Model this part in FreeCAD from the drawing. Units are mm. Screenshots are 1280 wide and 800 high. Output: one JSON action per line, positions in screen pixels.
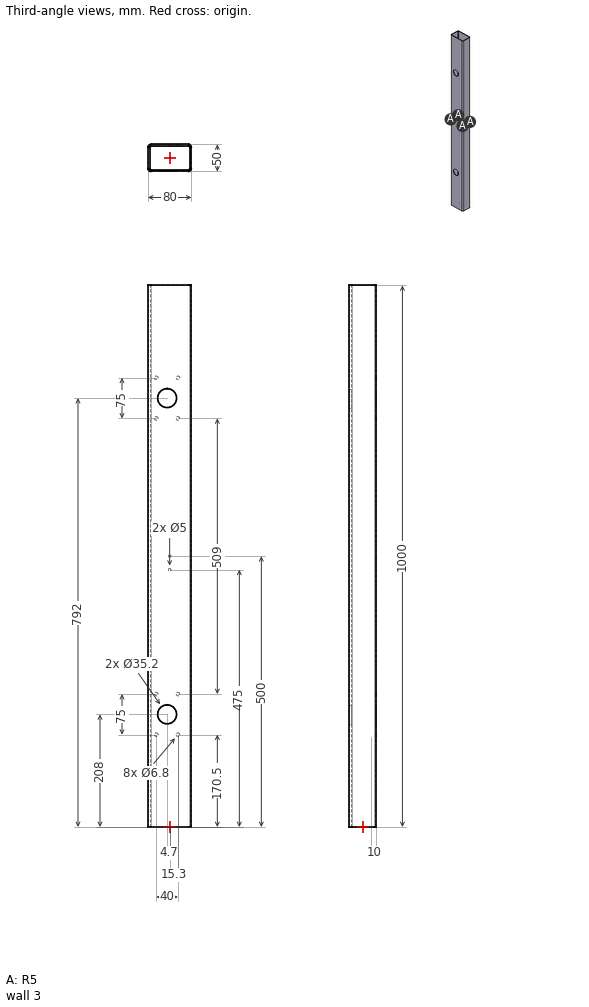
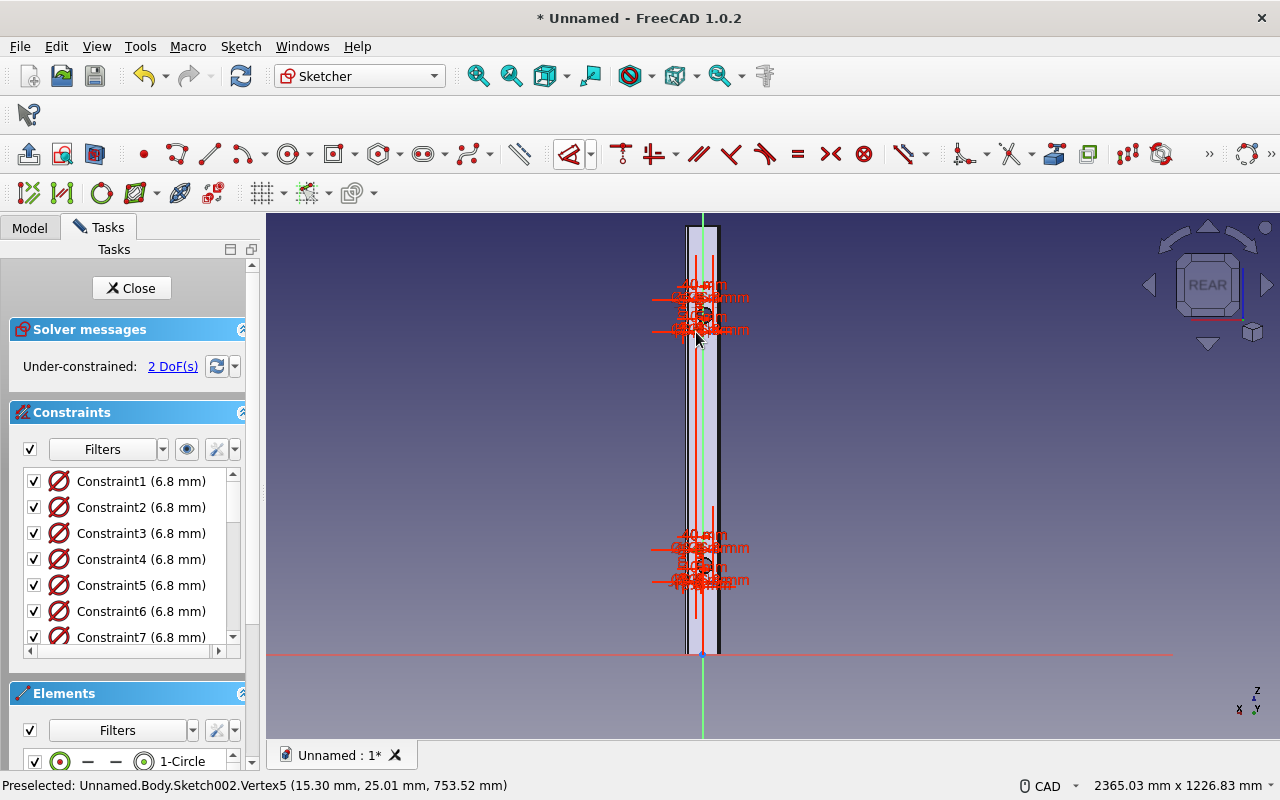
{"action": "key", "text": "i"}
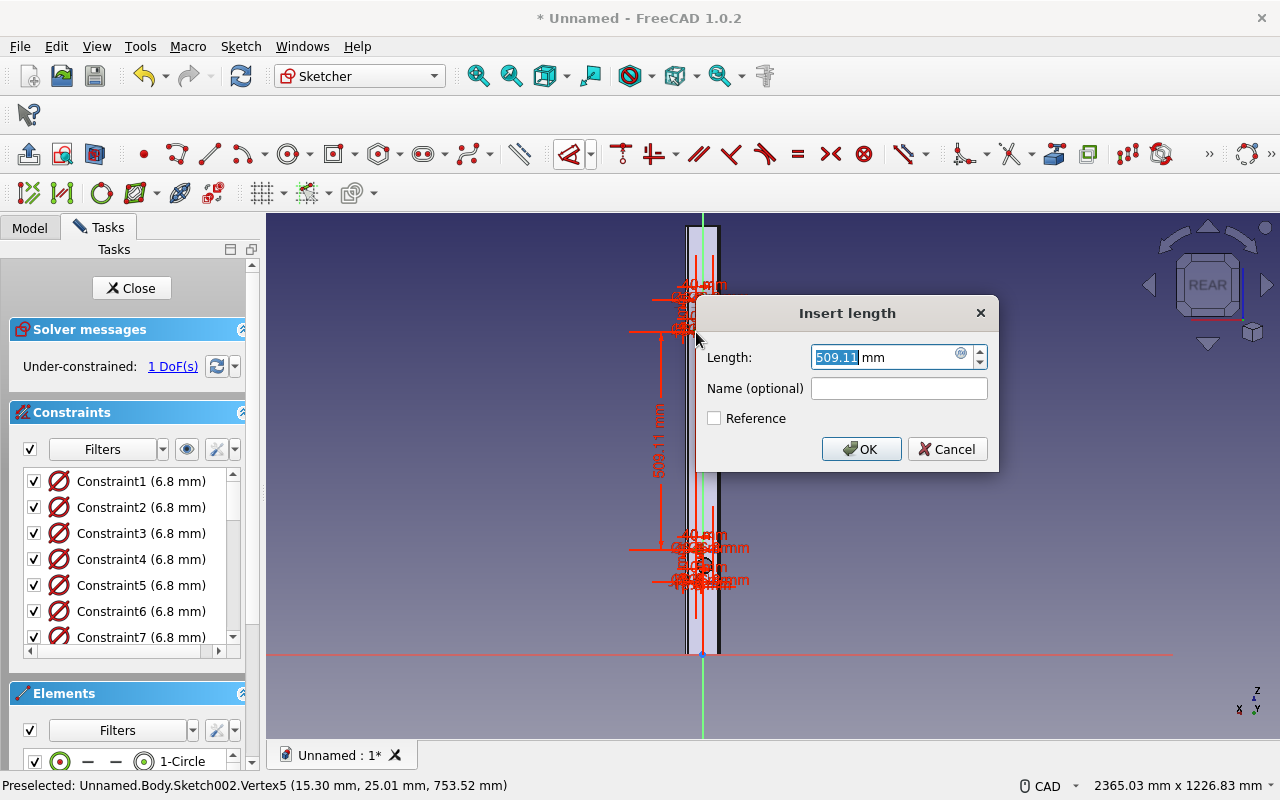
{"action": "type", "text": "509"}
{"action": "key", "text": "Return"}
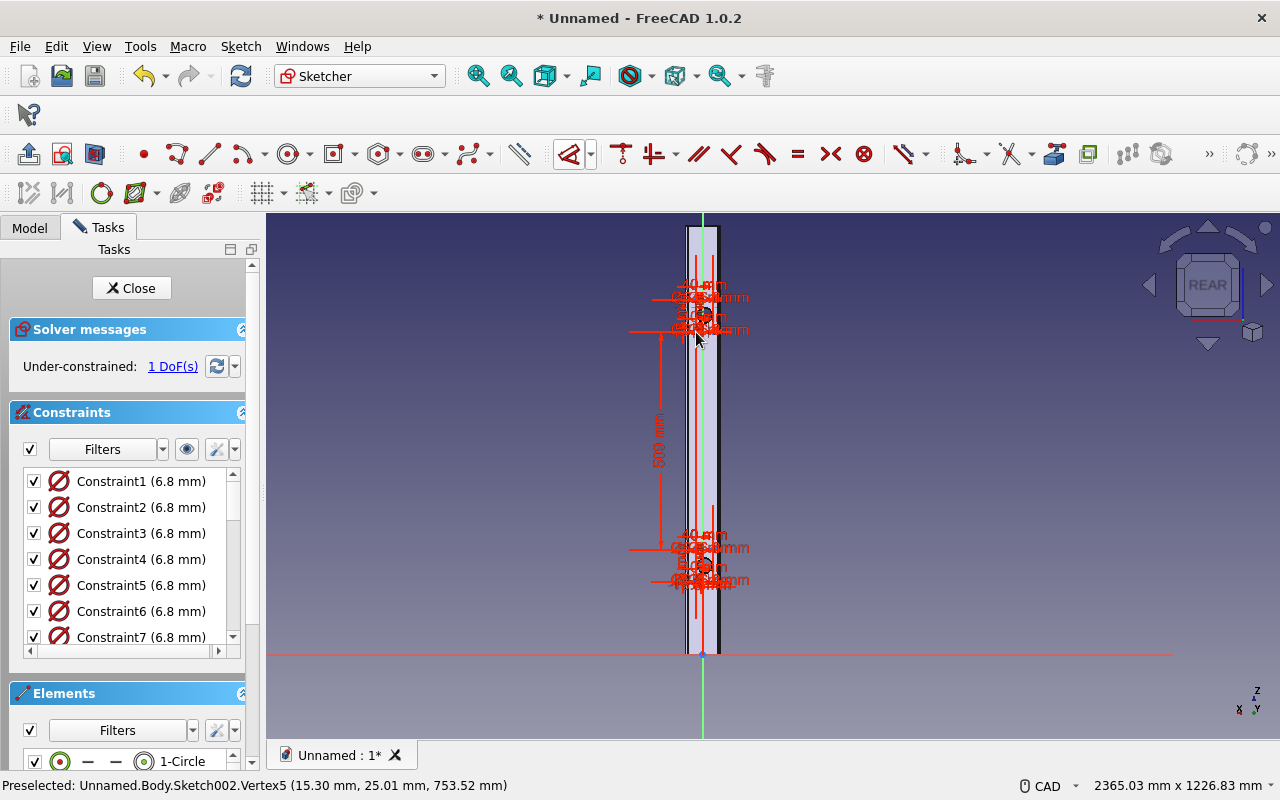
{"action": "left_click", "coordinate": [696, 582]}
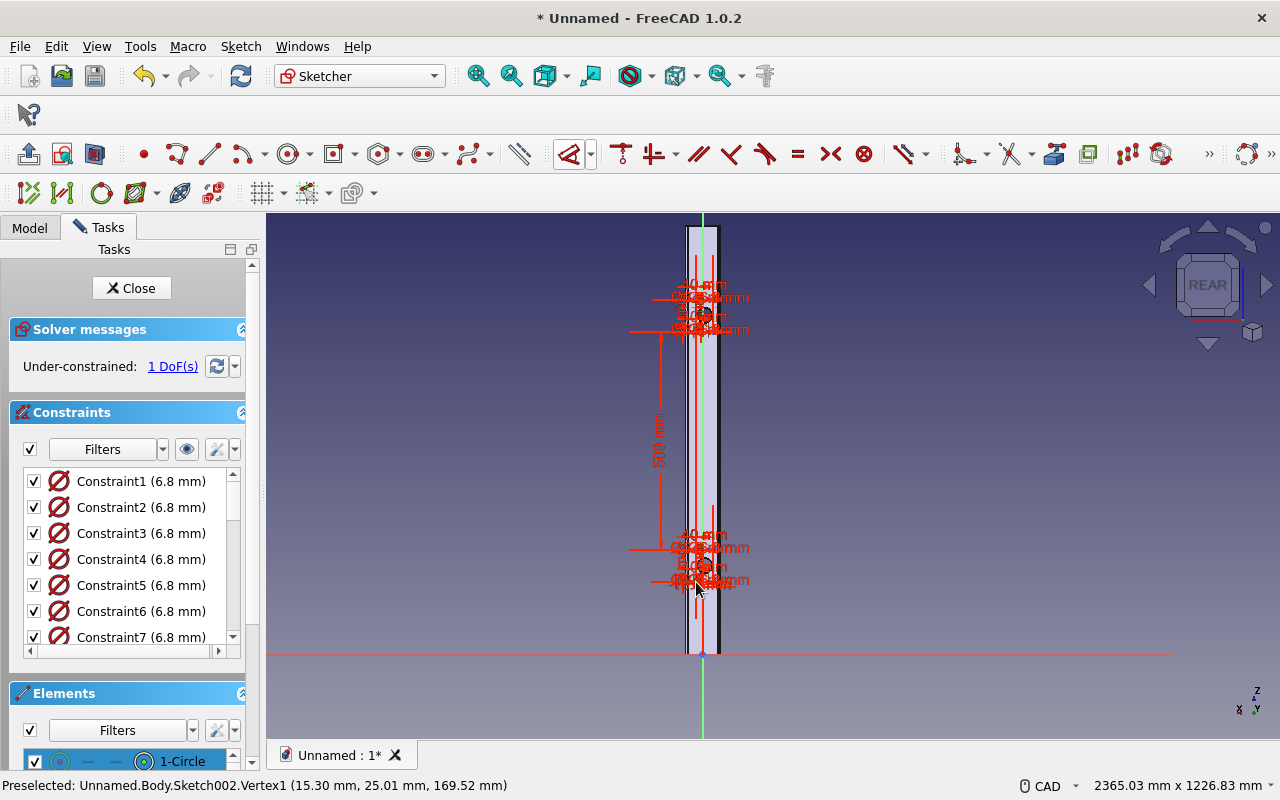
{"action": "left_click", "coordinate": [590, 154]}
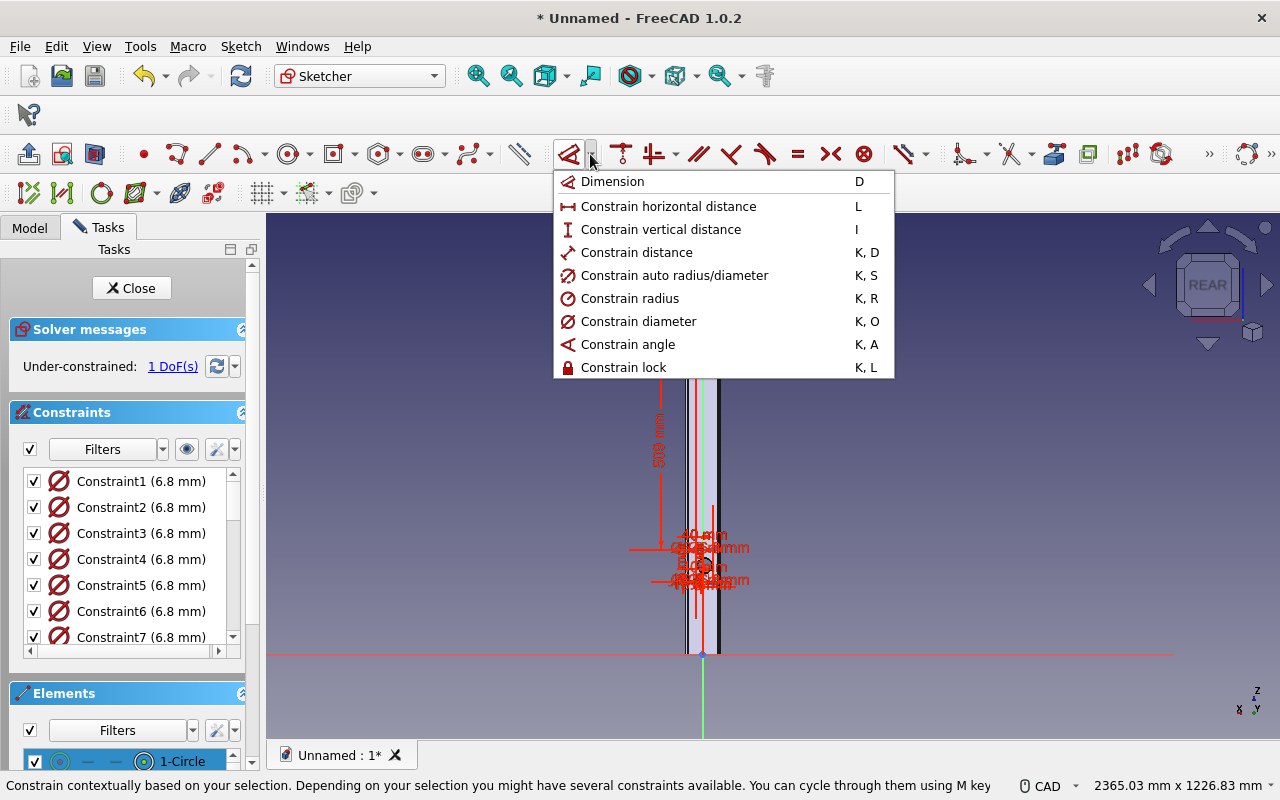
{"action": "left_click", "coordinate": [724, 230]}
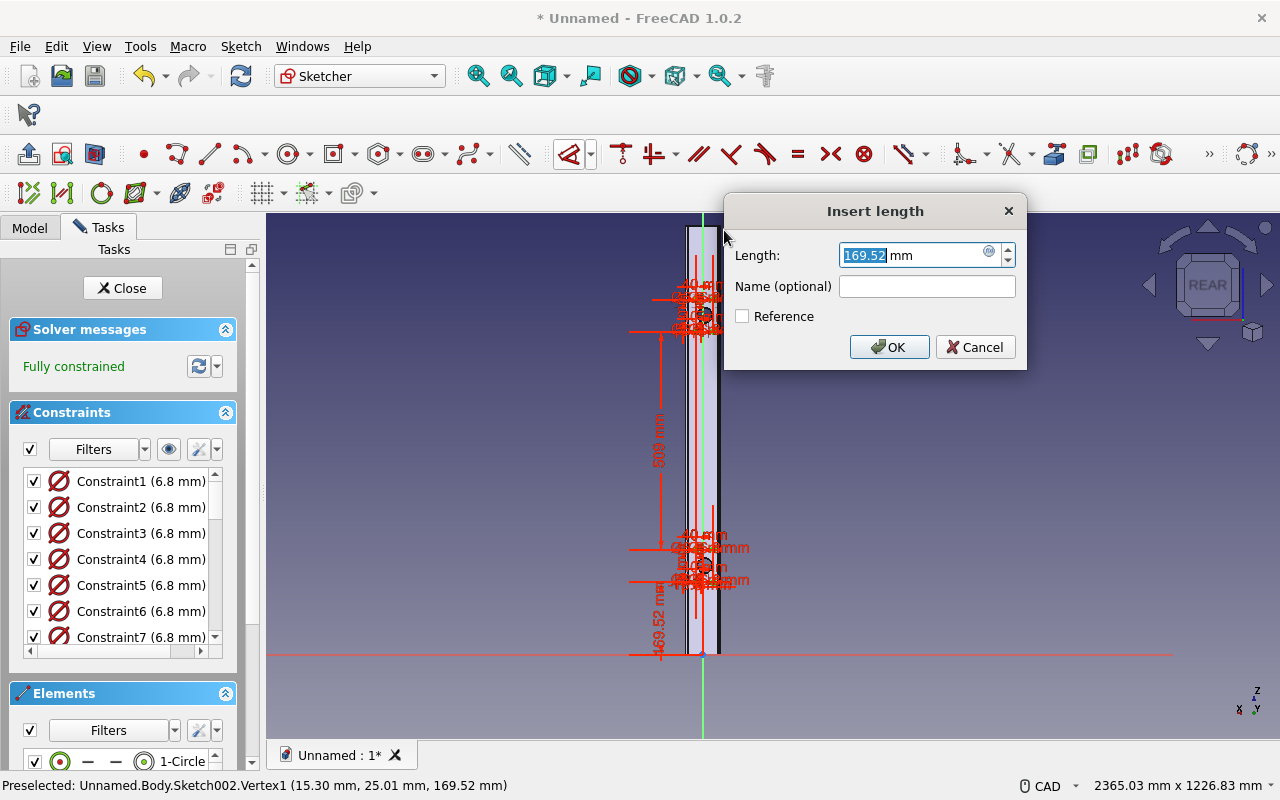
{"action": "type", "text": "170.5"}
{"action": "key", "text": "Return"}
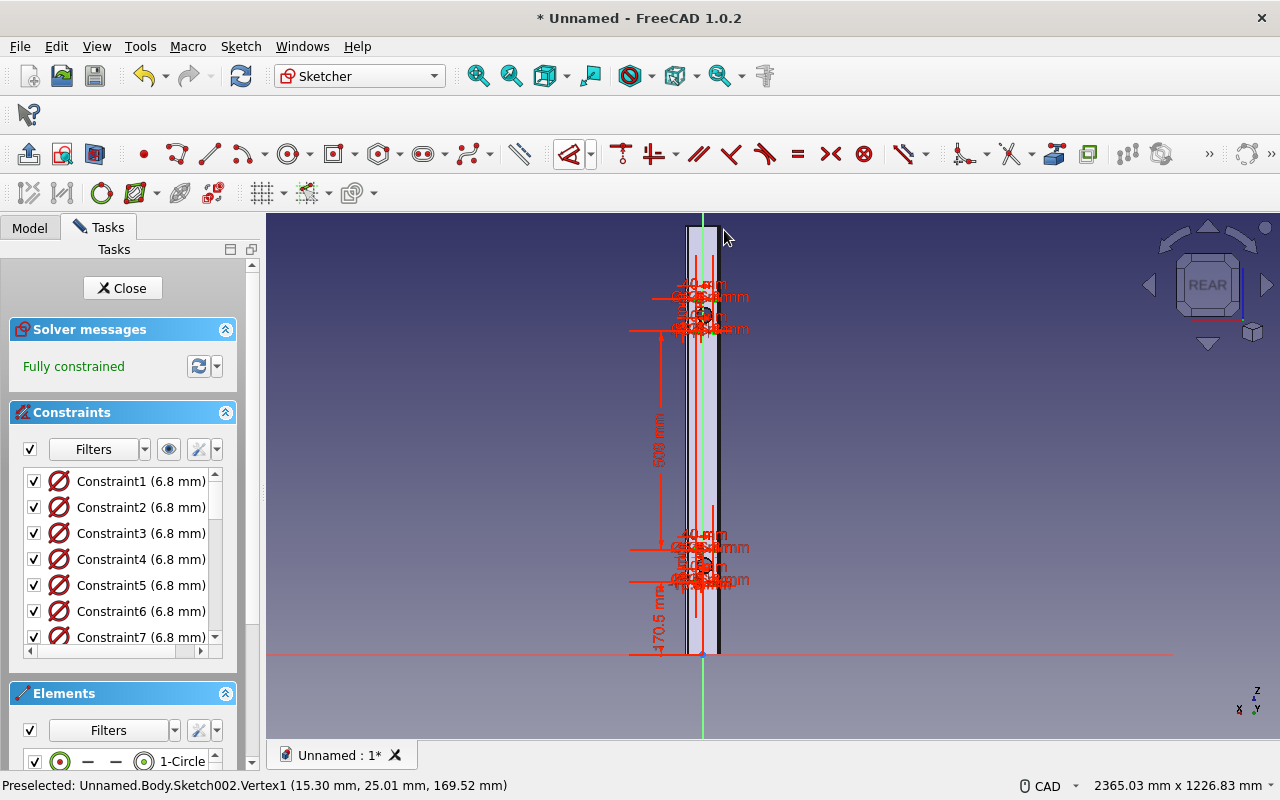
{"action": "left_click", "coordinate": [123, 288]}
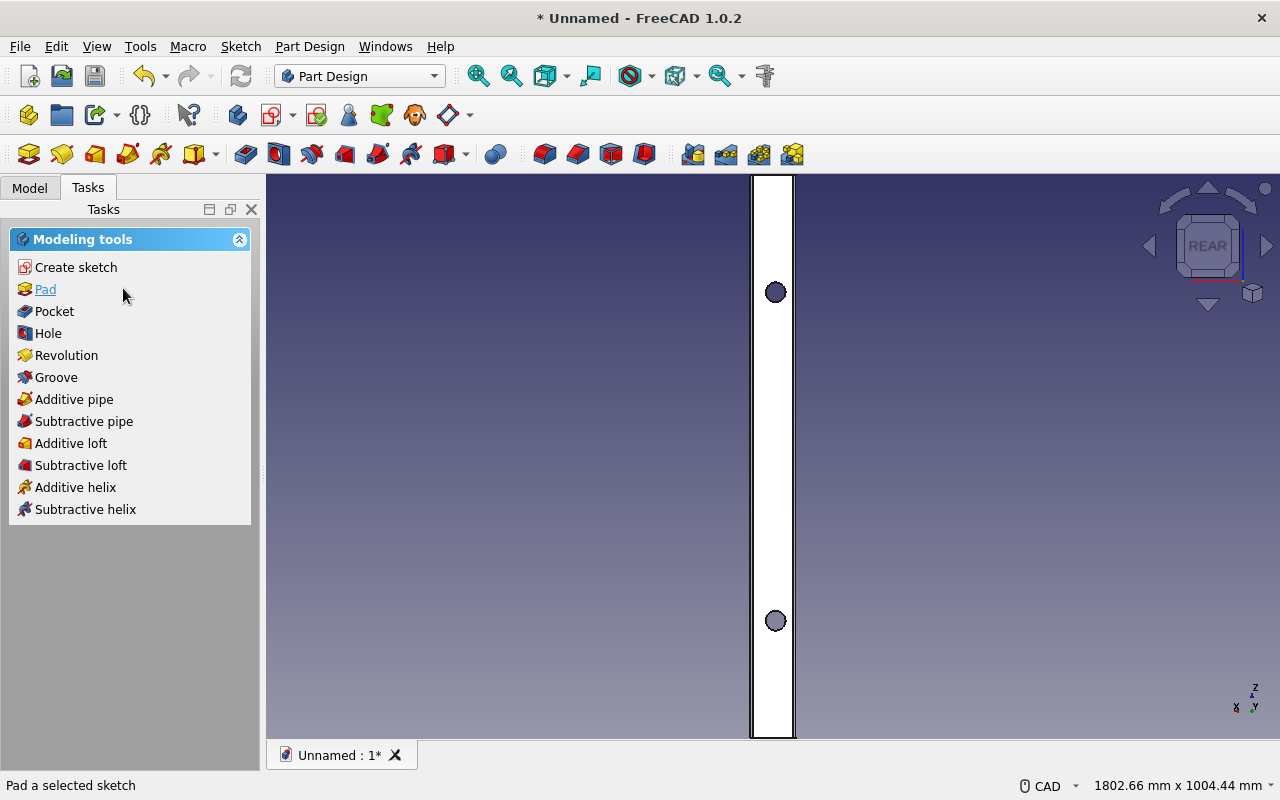
{"action": "left_click", "coordinate": [246, 154]}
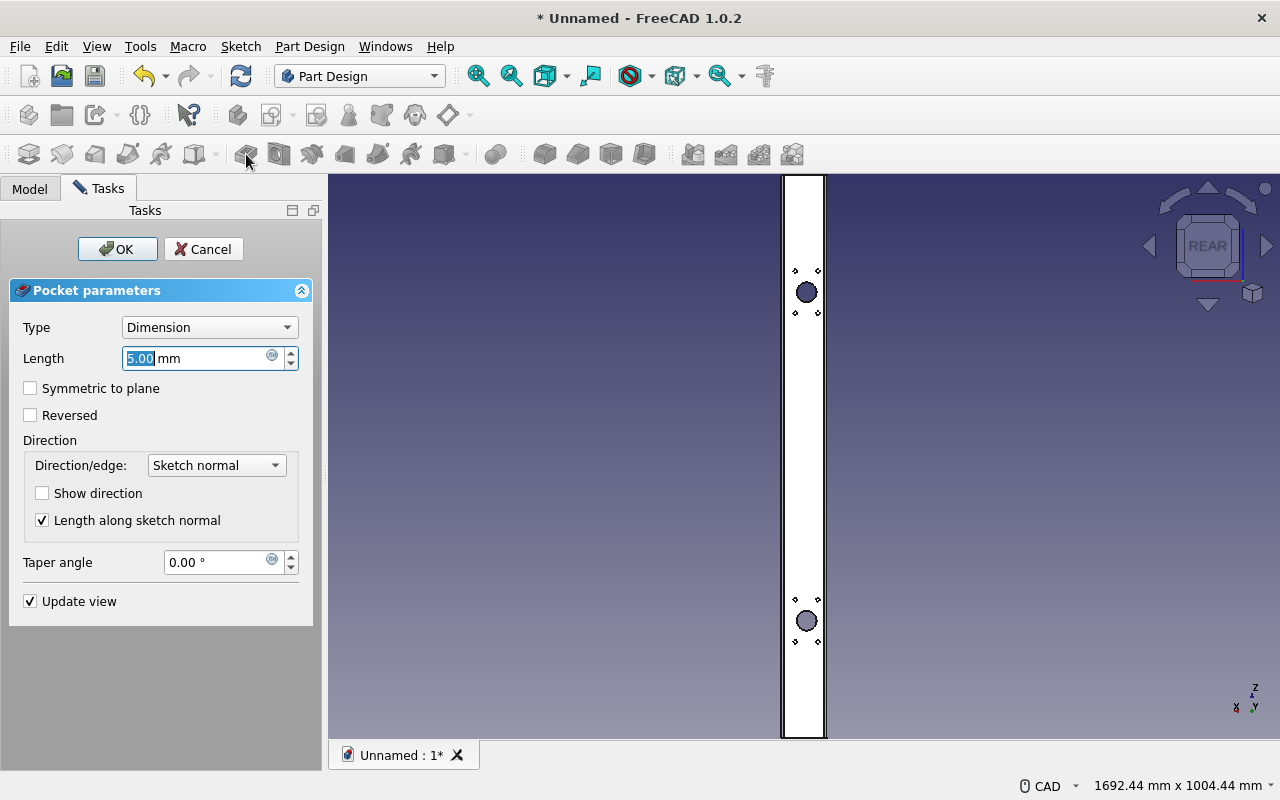
{"action": "type", "text": "10"}
{"action": "key", "text": "Tab"}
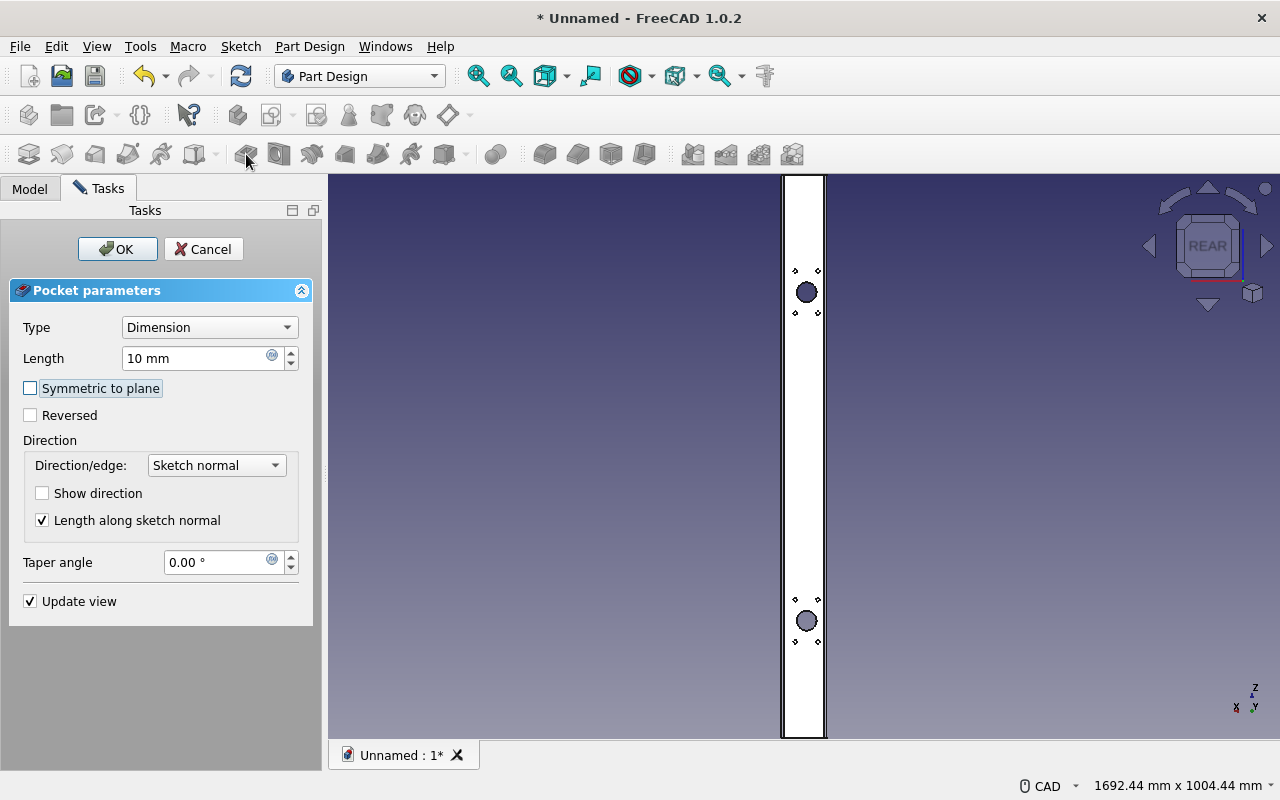
{"action": "left_click", "coordinate": [118, 249]}